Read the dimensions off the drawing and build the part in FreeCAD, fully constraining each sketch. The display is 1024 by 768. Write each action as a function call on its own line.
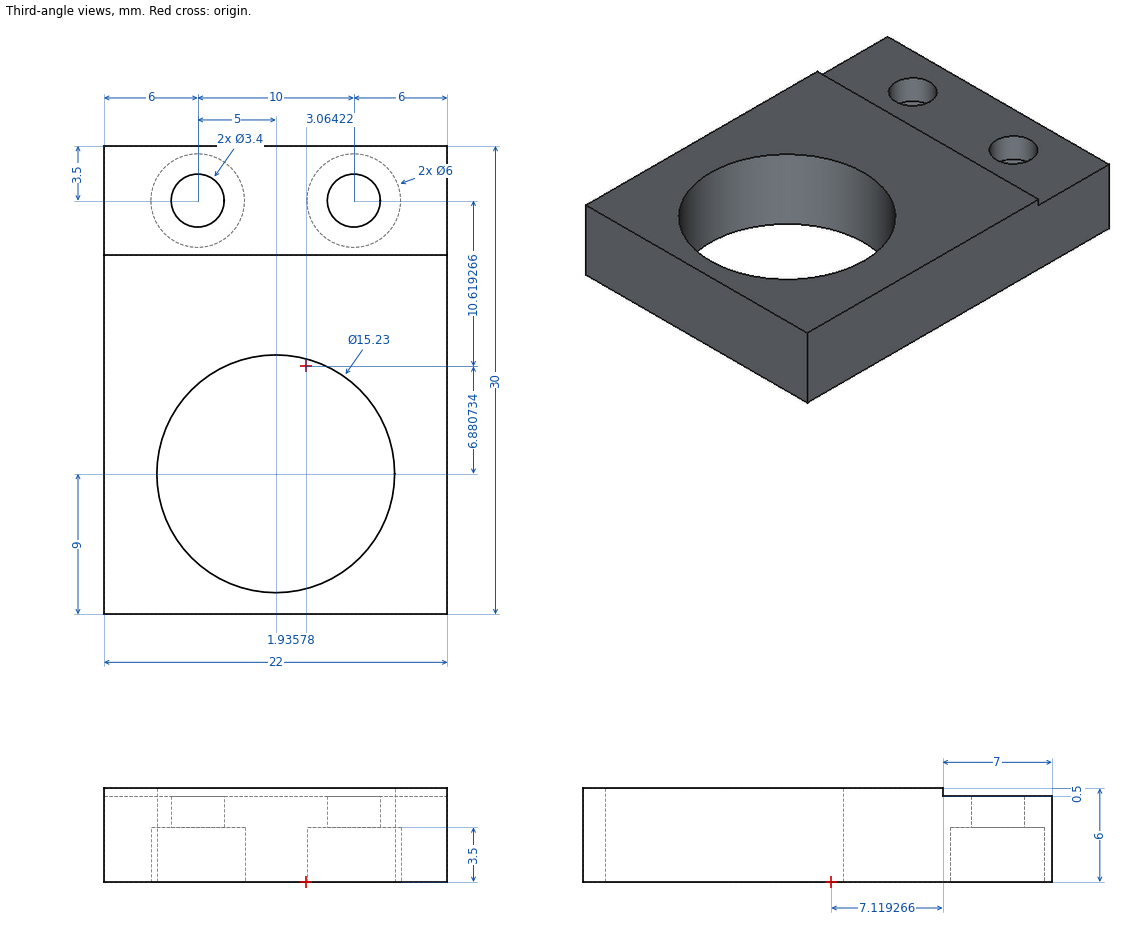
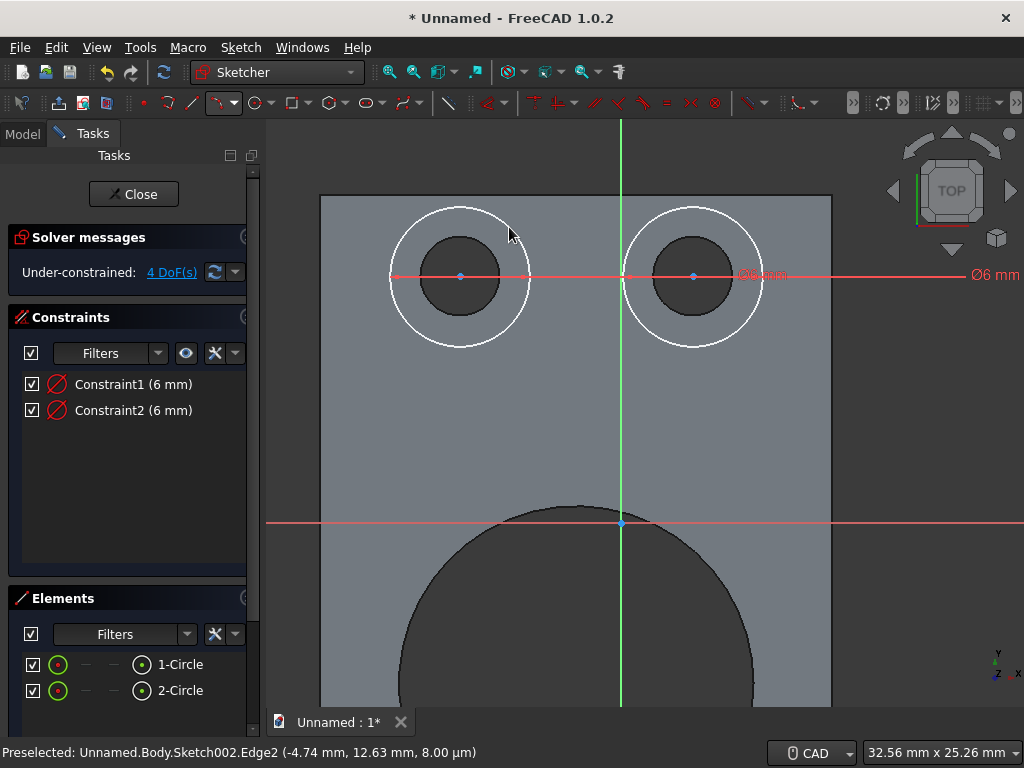
click(693, 277)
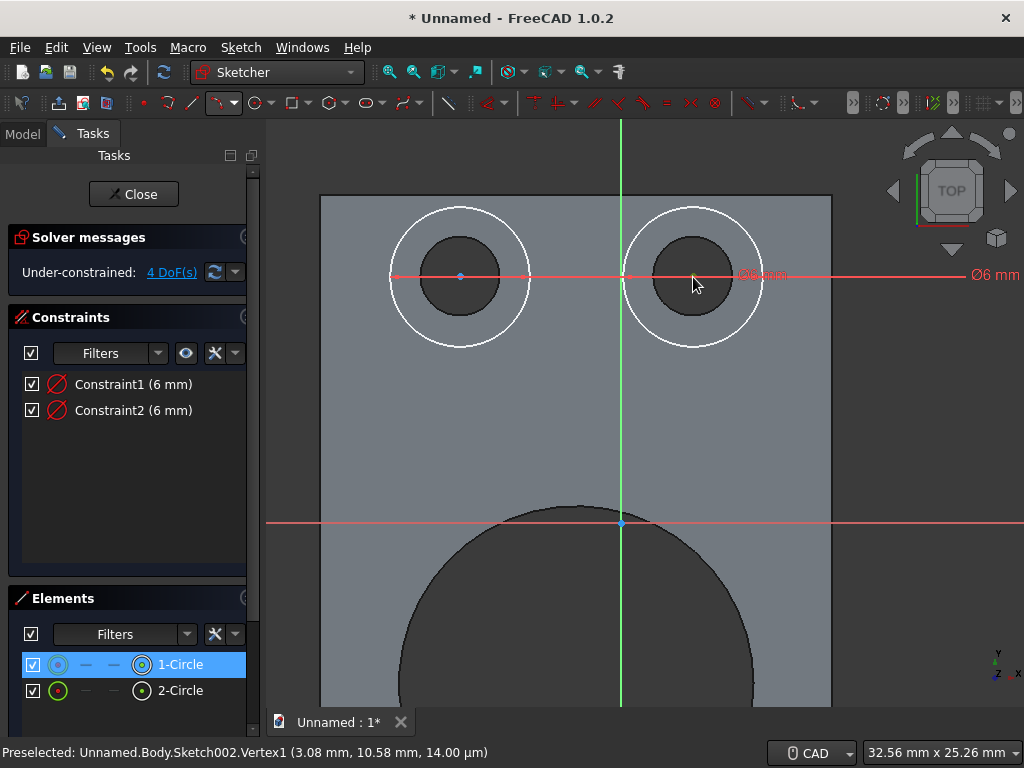
click(460, 277)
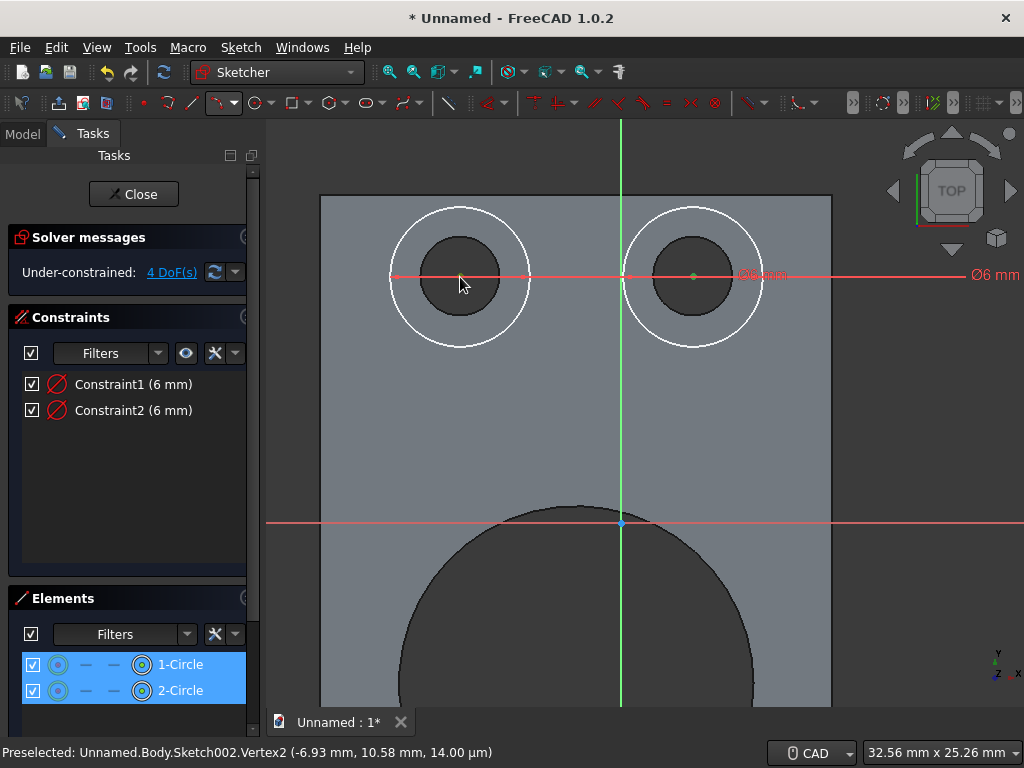
key(h)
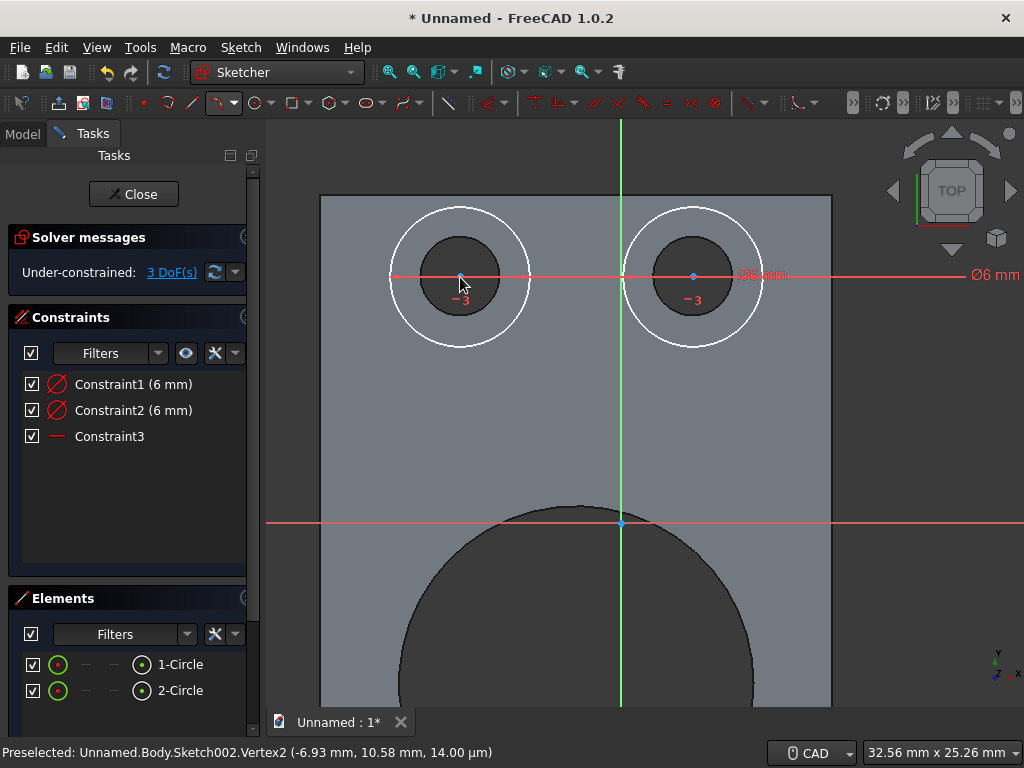
click(693, 277)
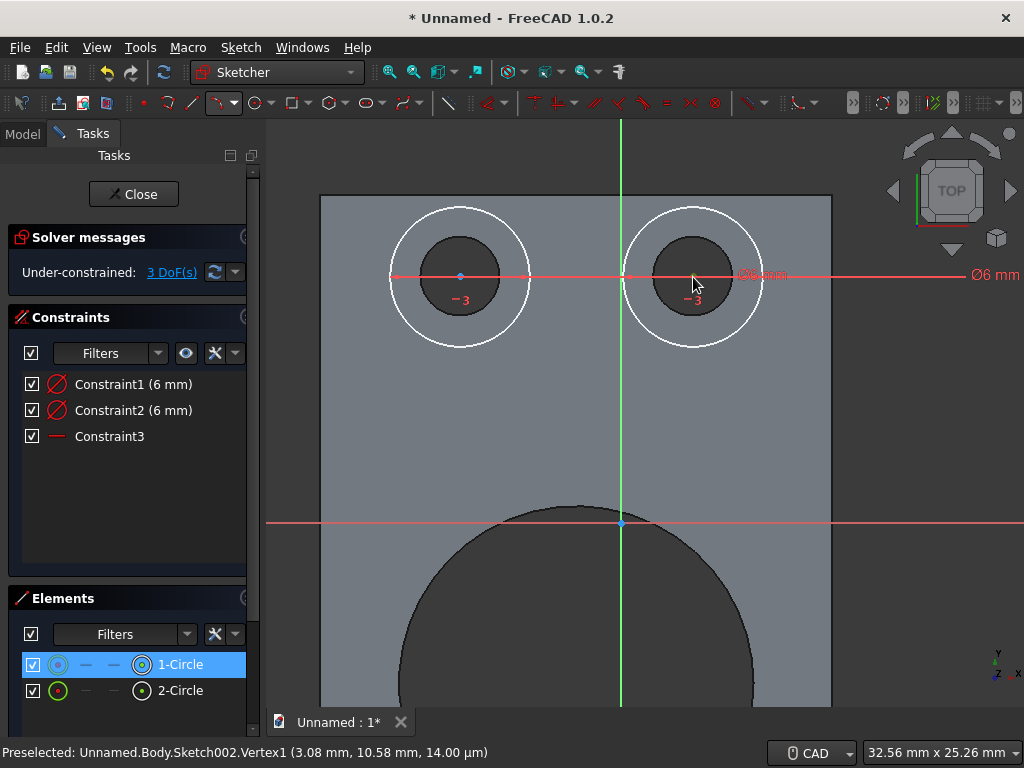
click(460, 277)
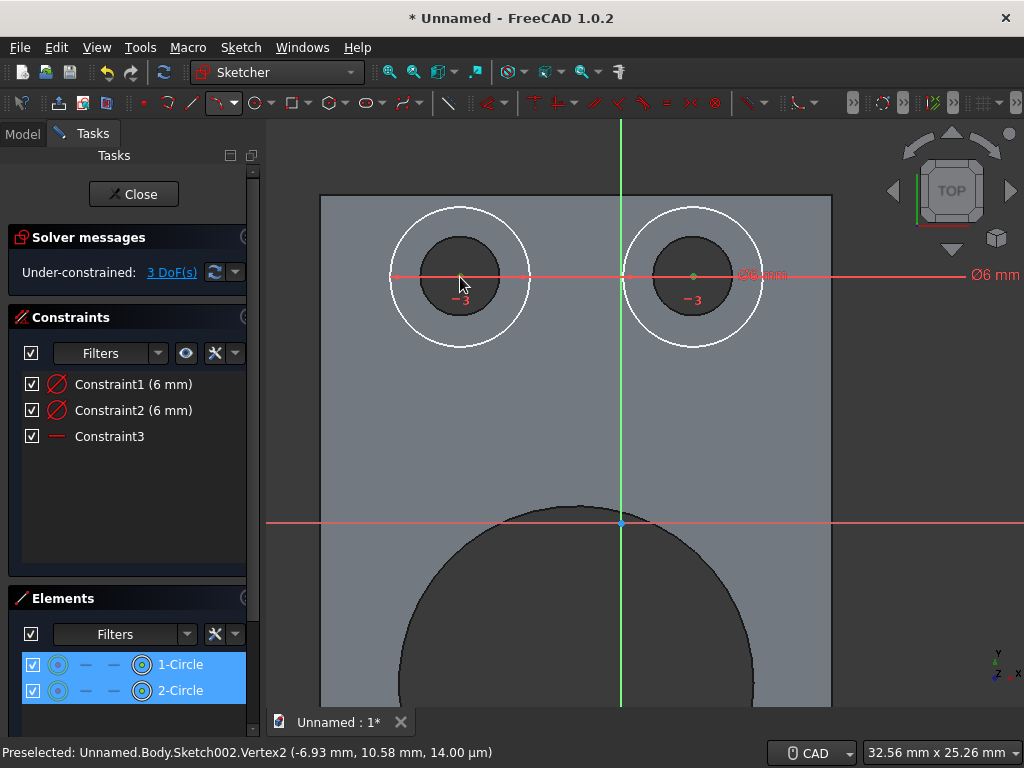
key(l)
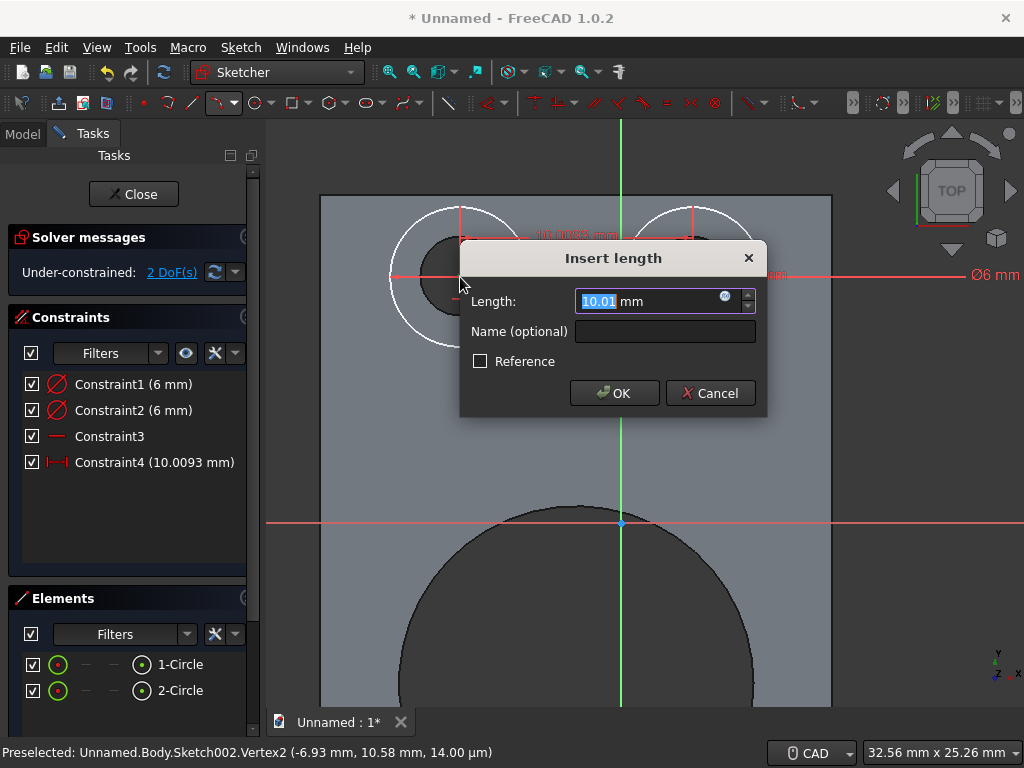
text(10)
key(Return)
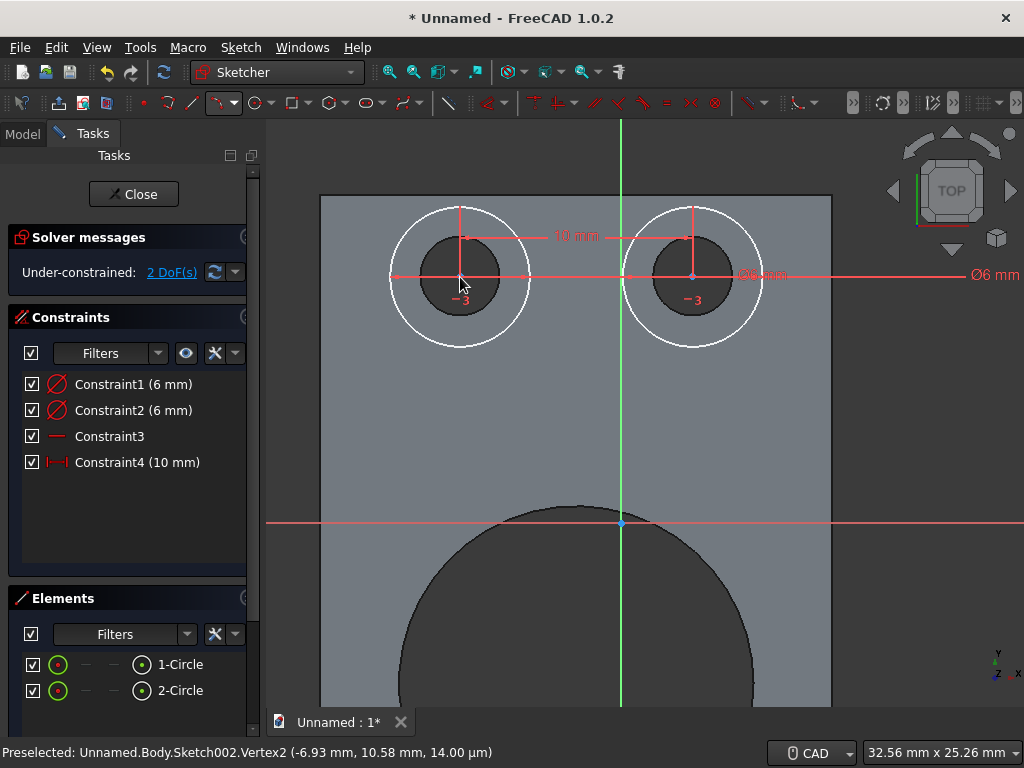
click(693, 277)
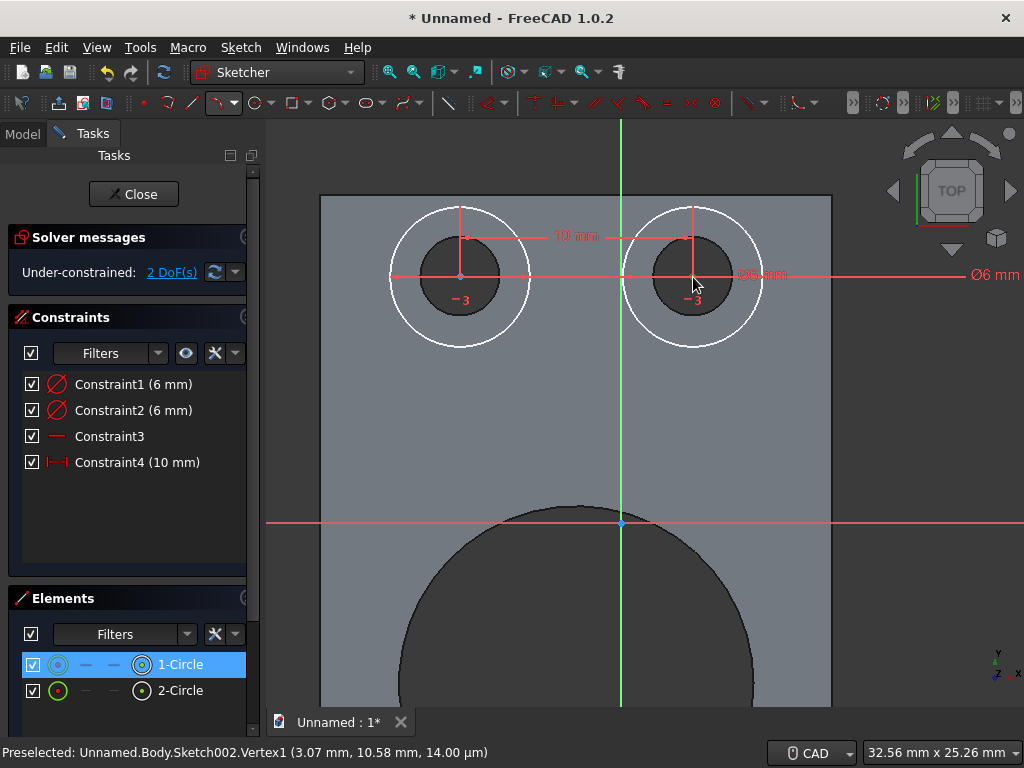
key(l)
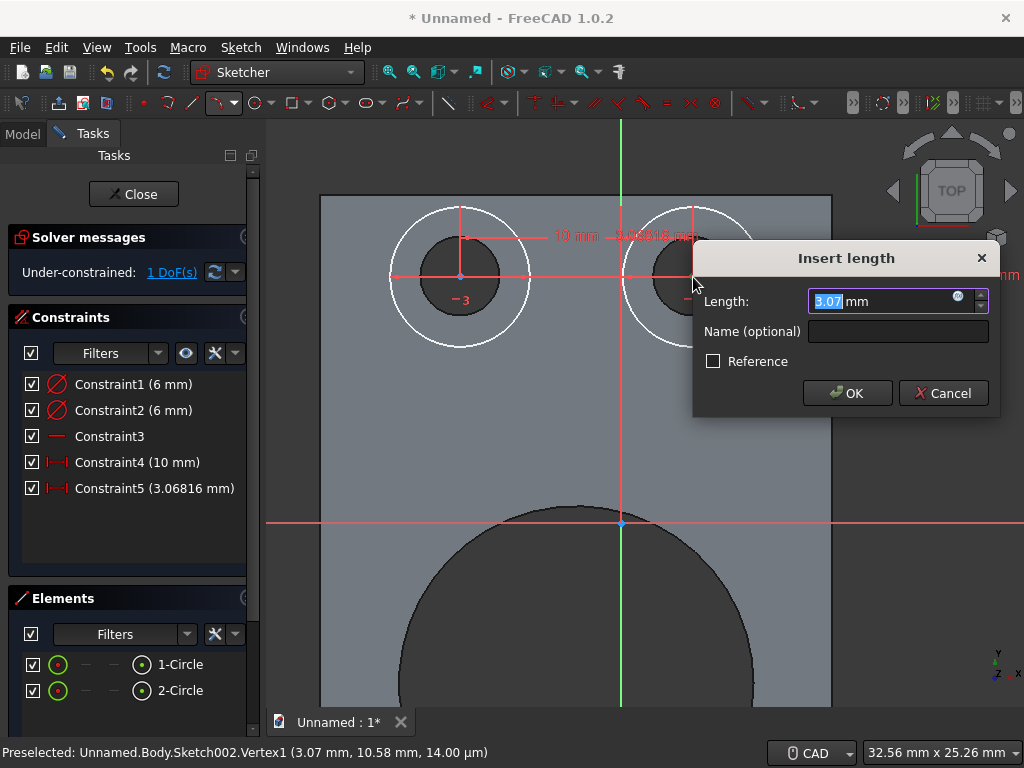
text(3.06422)
key(Return)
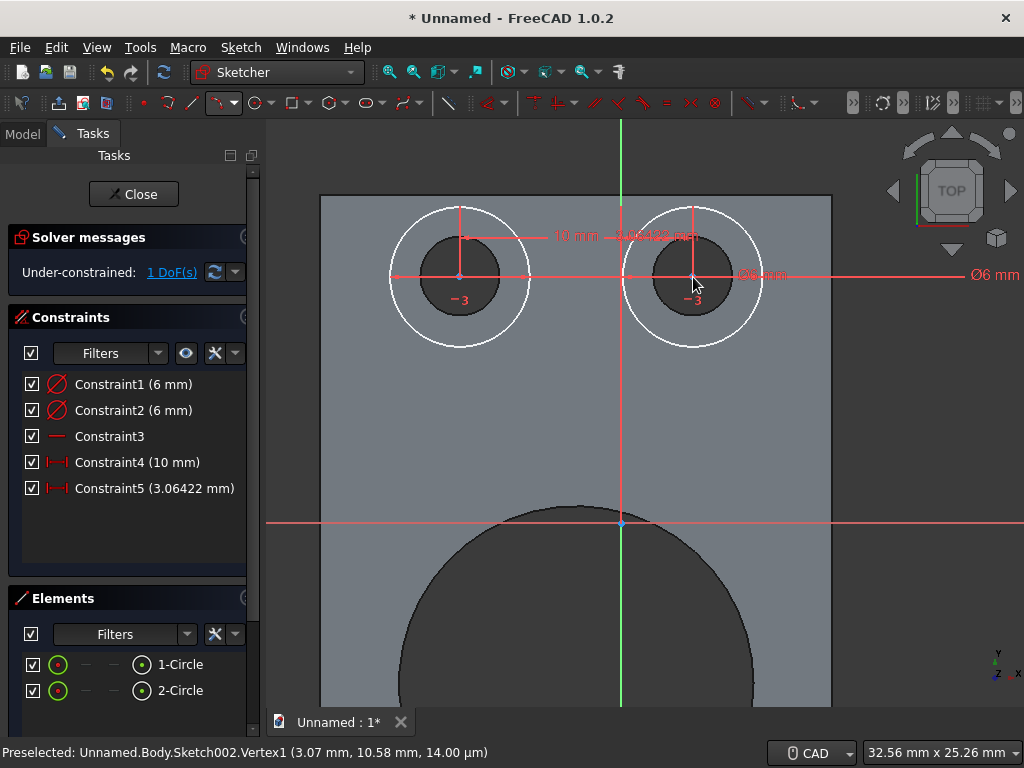
click(693, 277)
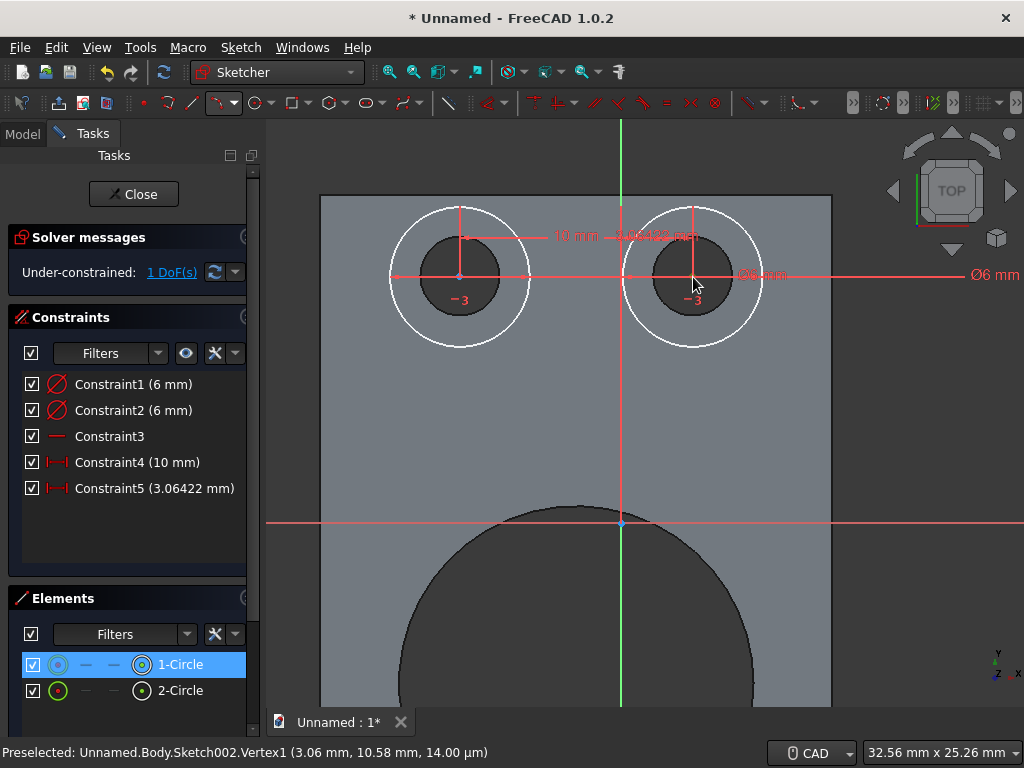
click(506, 104)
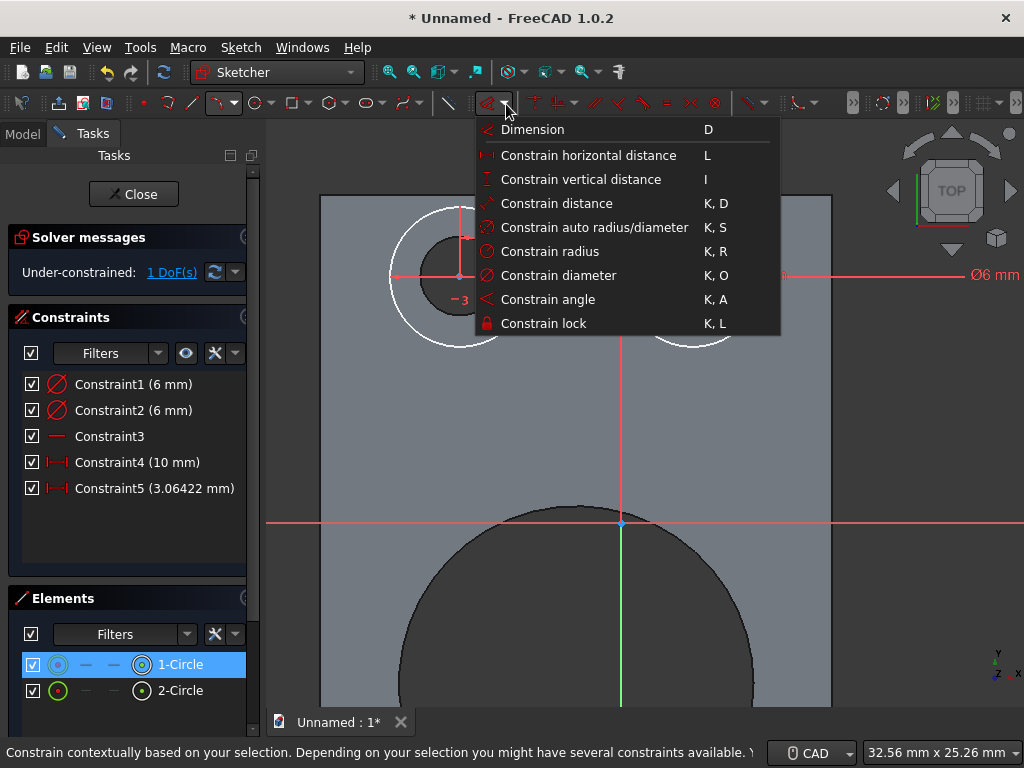
click(628, 179)